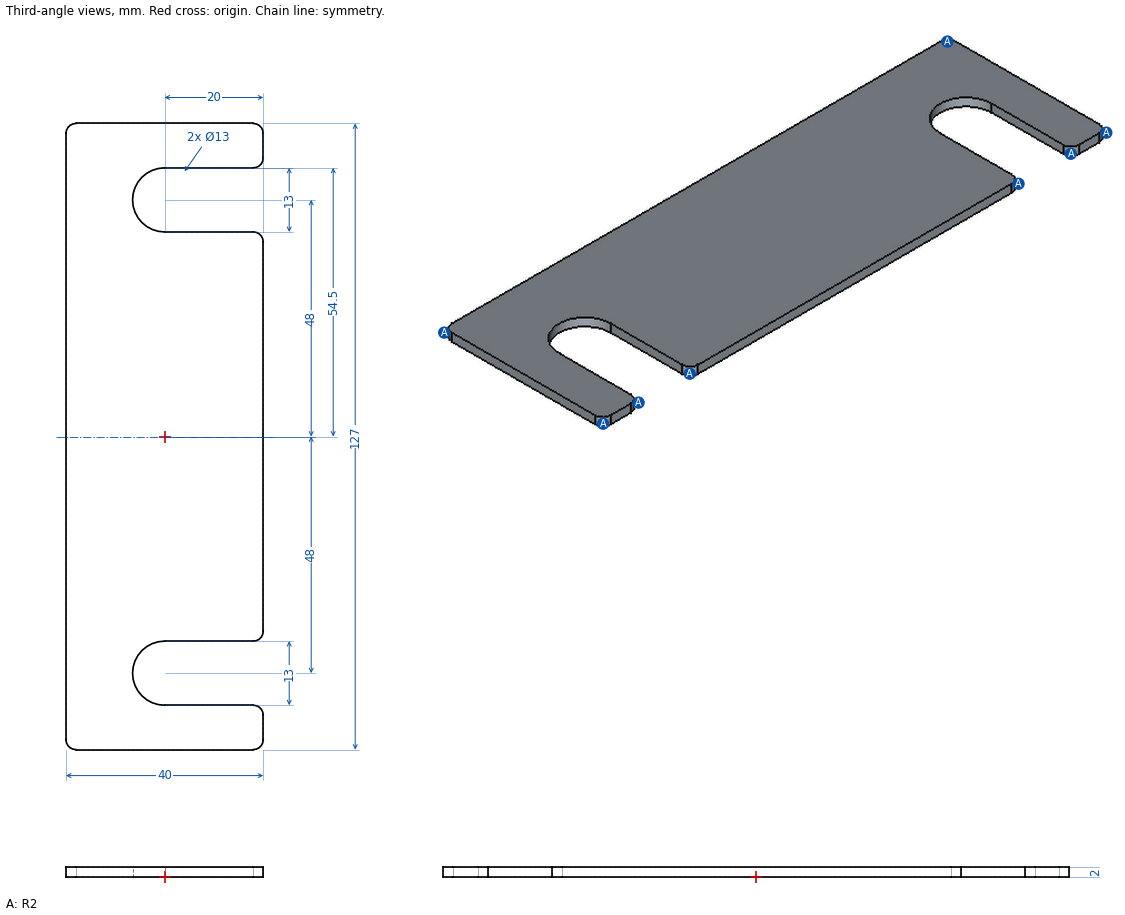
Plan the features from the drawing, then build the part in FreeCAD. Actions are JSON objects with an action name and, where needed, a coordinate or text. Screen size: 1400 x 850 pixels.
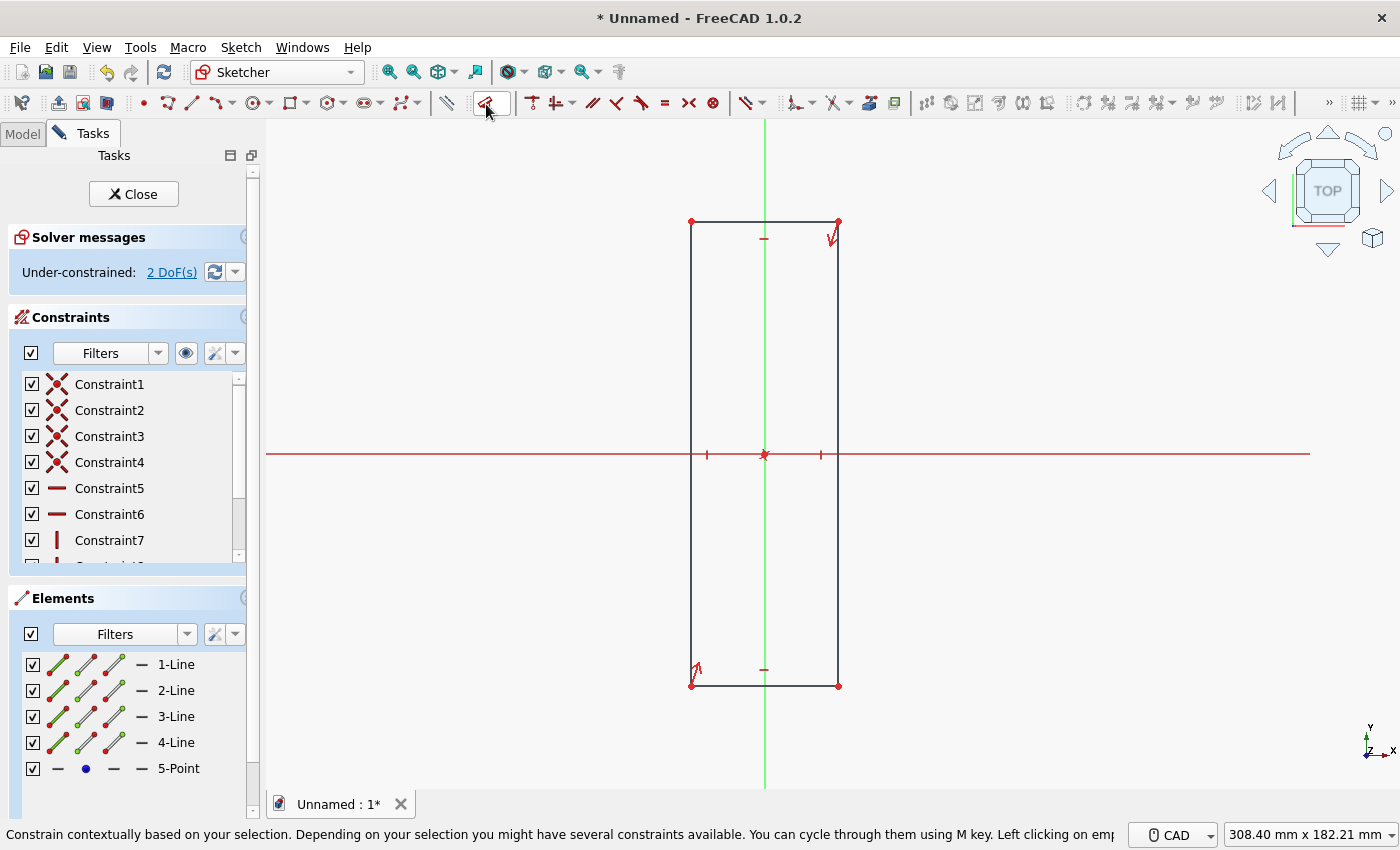
{"action": "left_click", "coordinate": [735, 686]}
{"action": "left_click", "coordinate": [731, 720]}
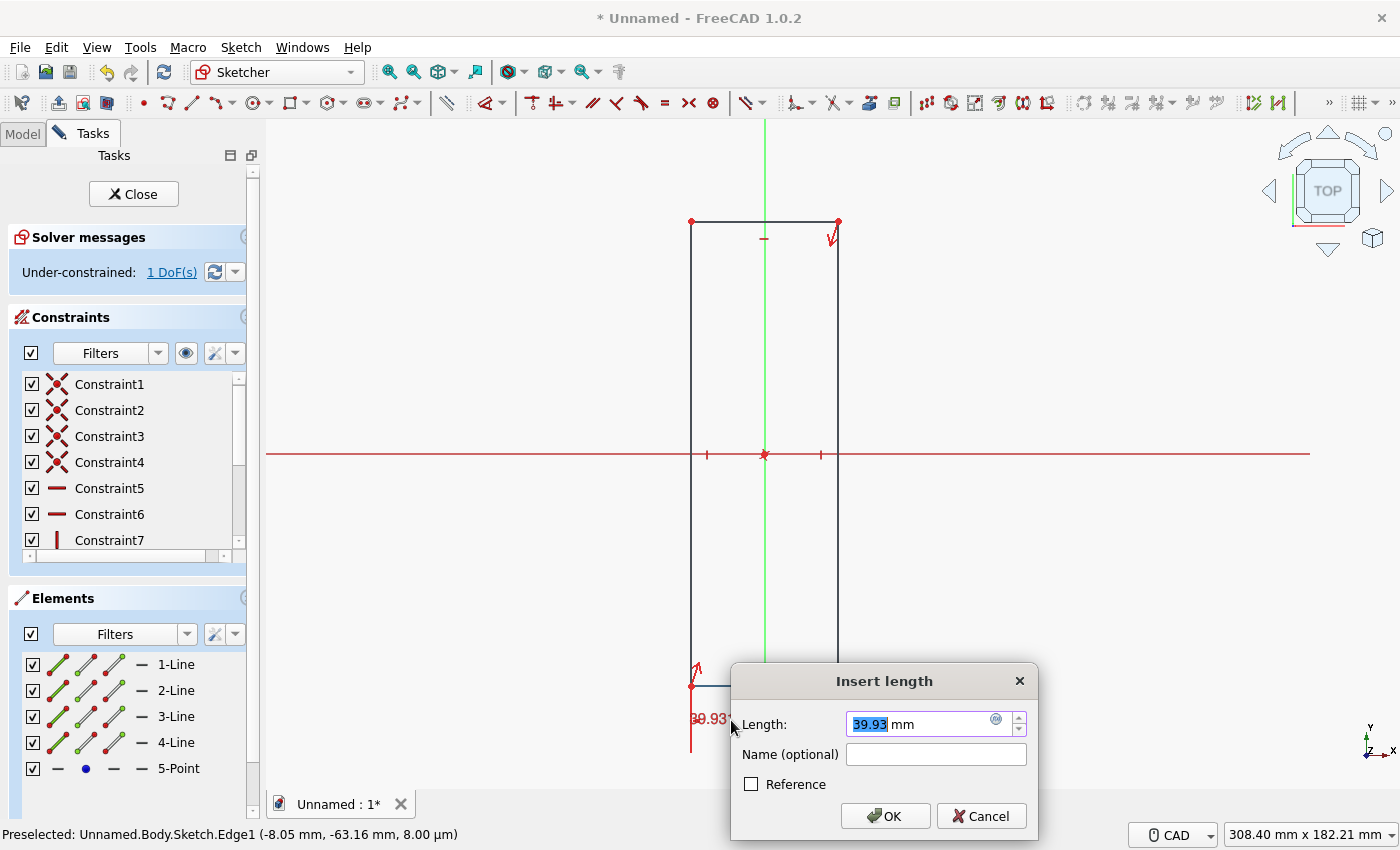
{"action": "type", "text": "40"}
{"action": "key", "text": "Return"}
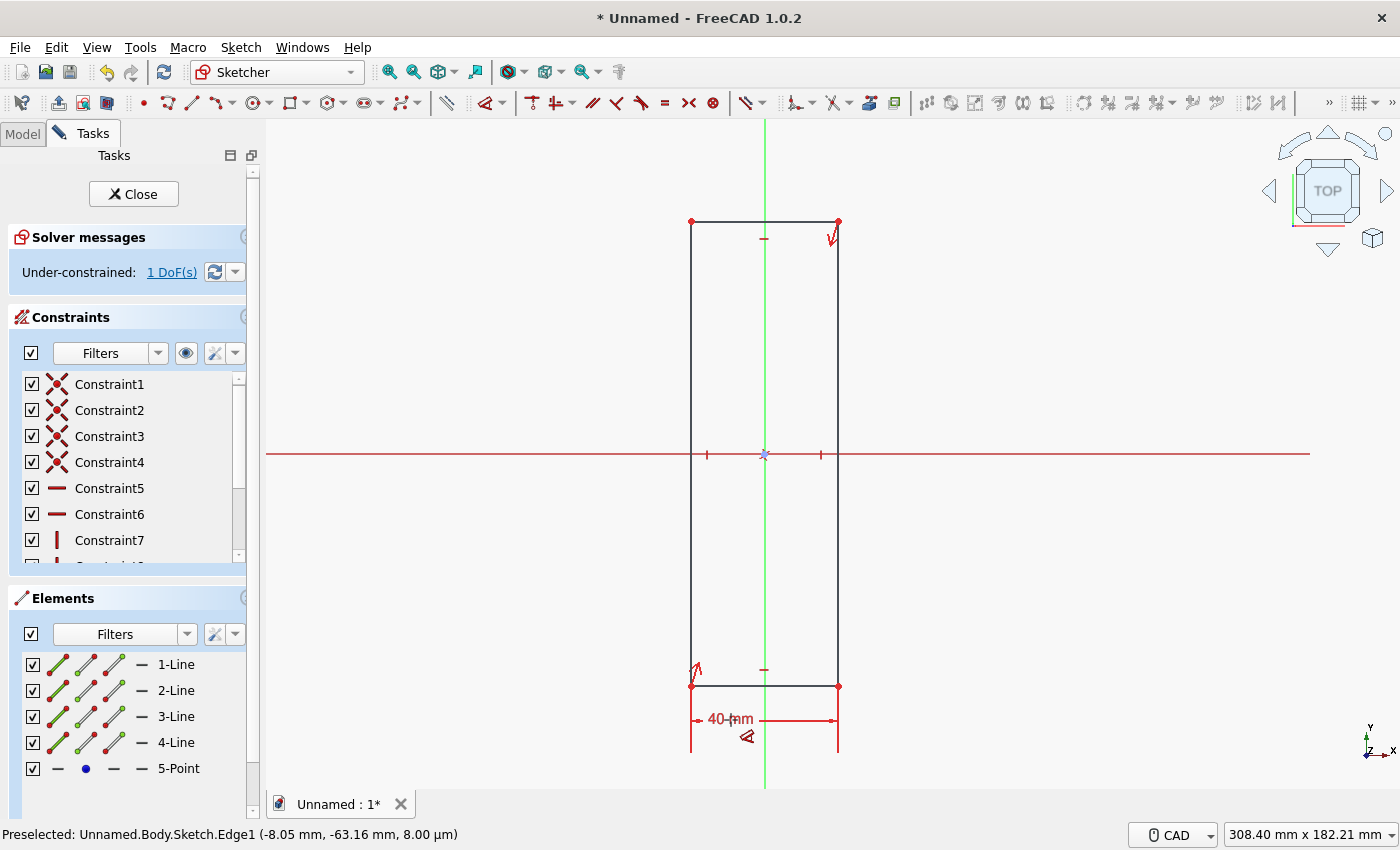
{"action": "left_click", "coordinate": [838, 547]}
{"action": "left_click", "coordinate": [872, 347]}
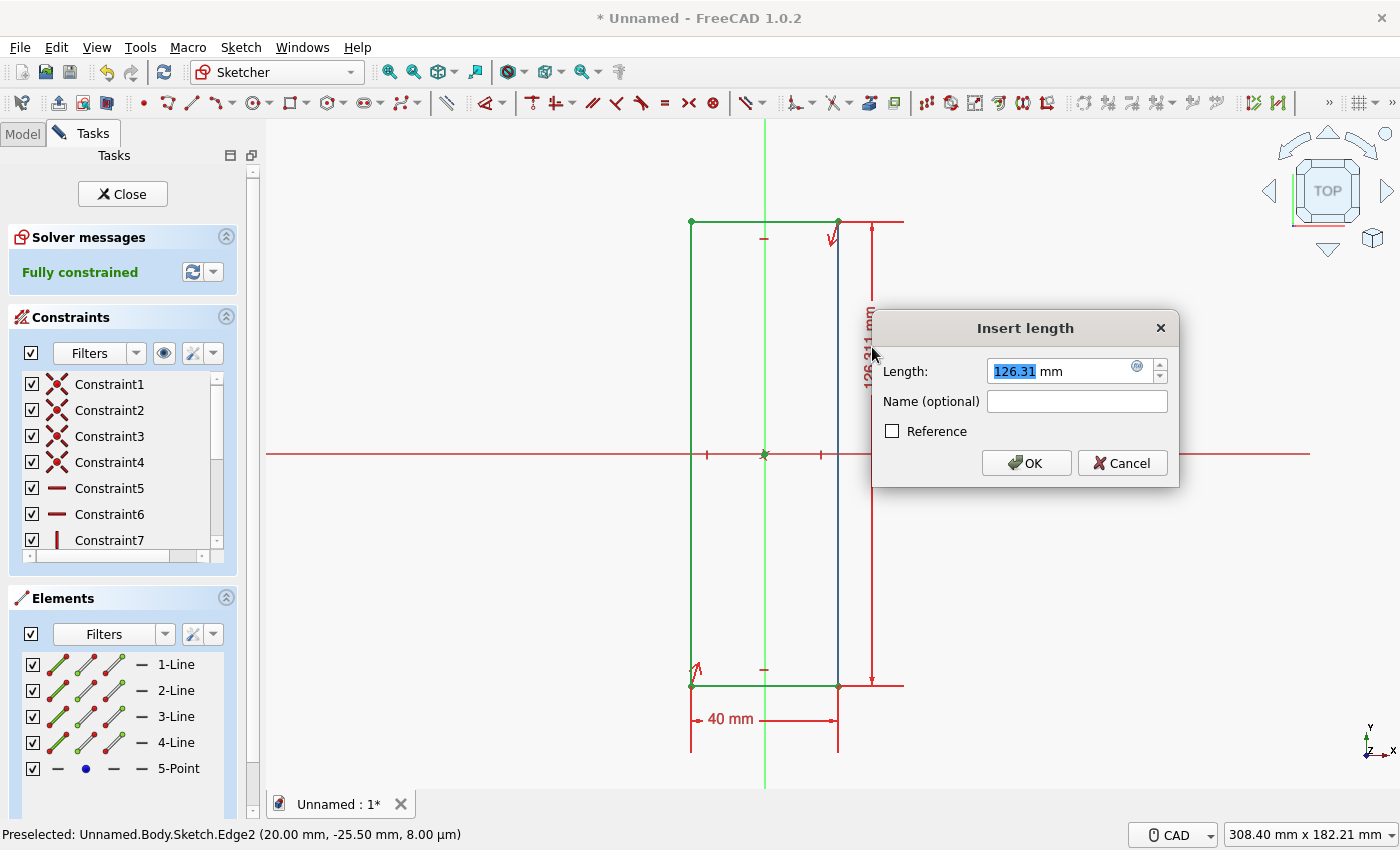
{"action": "type", "text": "127"}
{"action": "key", "text": "Return"}
{"action": "key", "text": "Escape"}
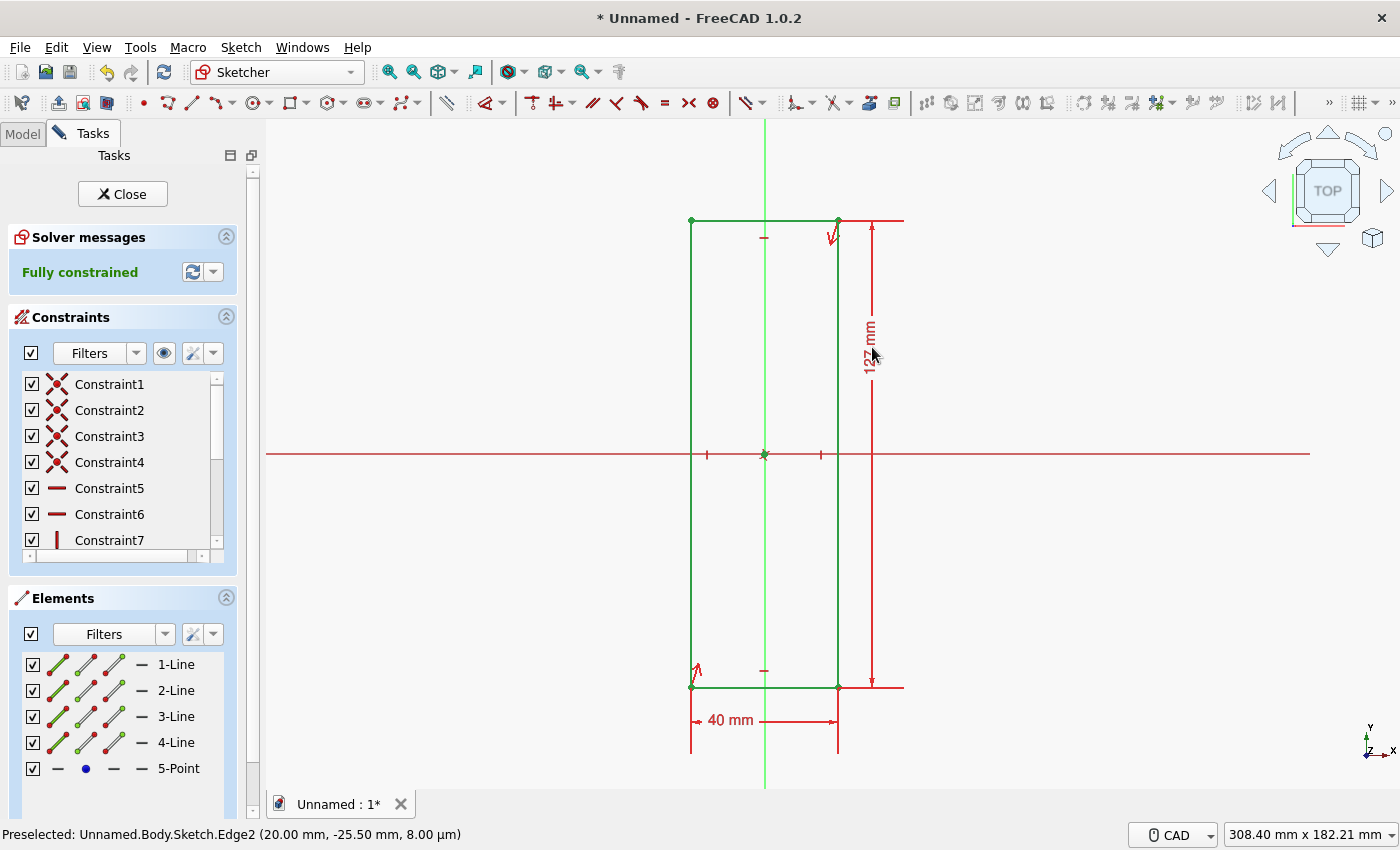
{"action": "left_click", "coordinate": [123, 194]}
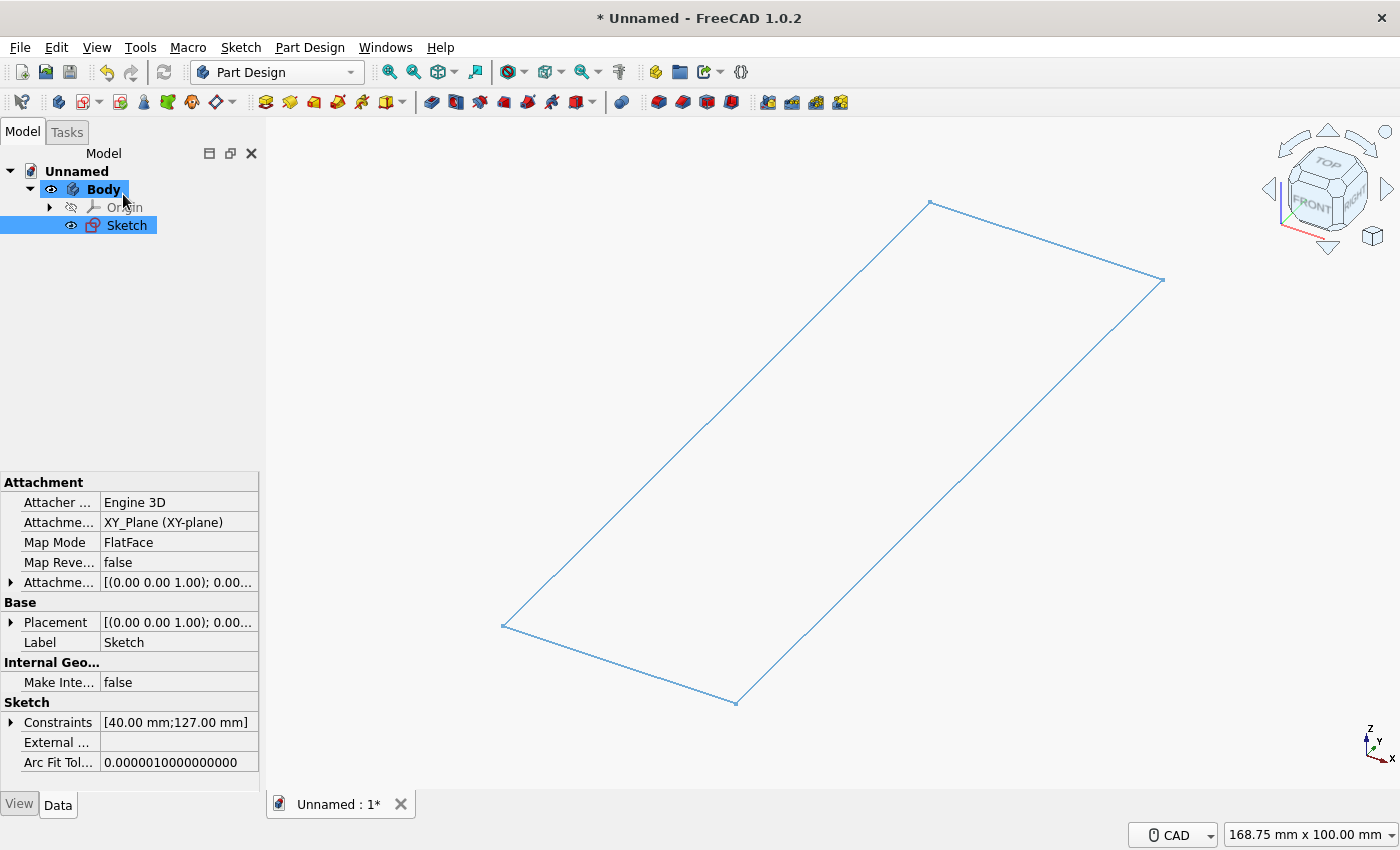
{"action": "left_click", "coordinate": [266, 102]}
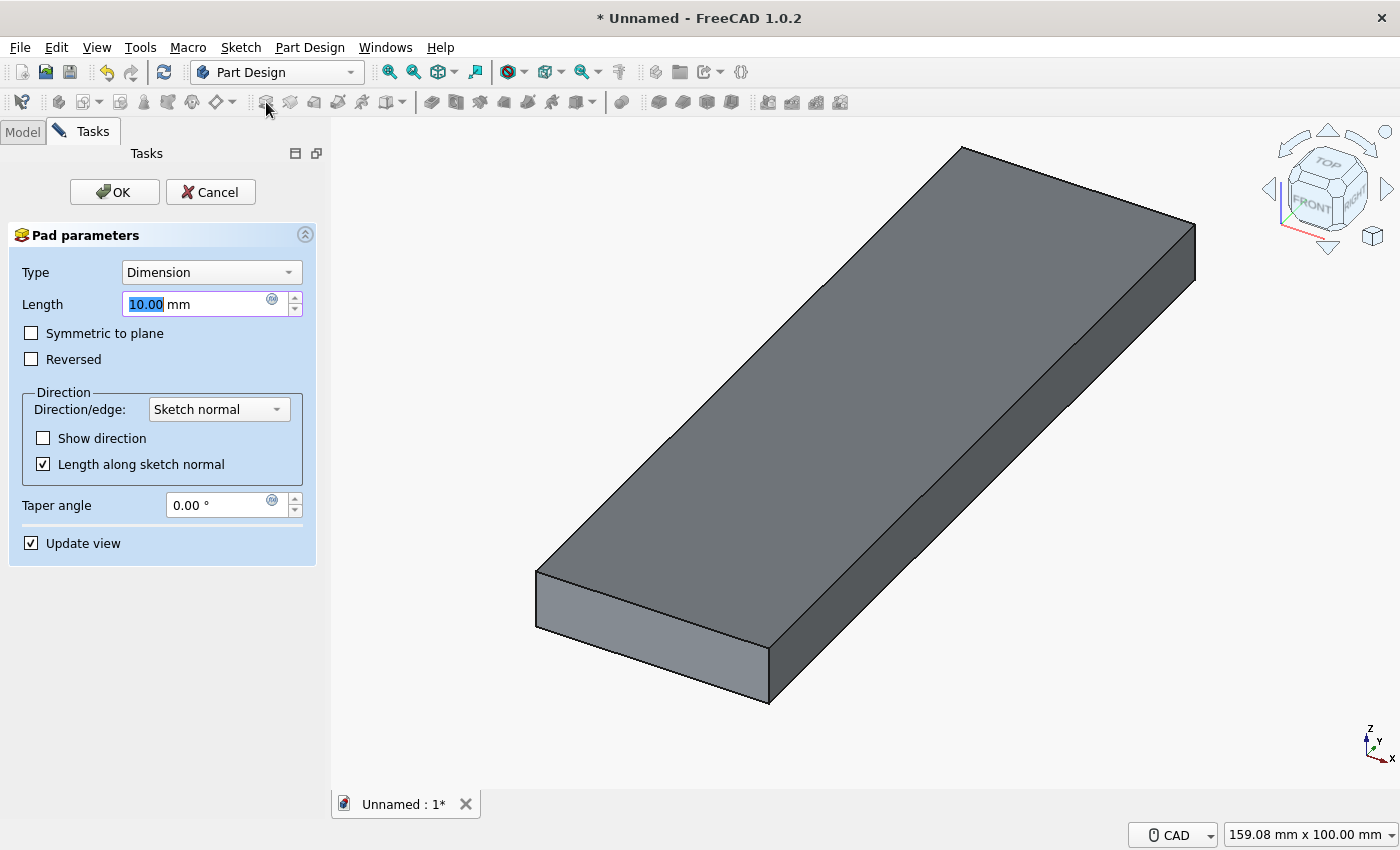
{"action": "type", "text": "2"}
{"action": "key", "text": "Tab"}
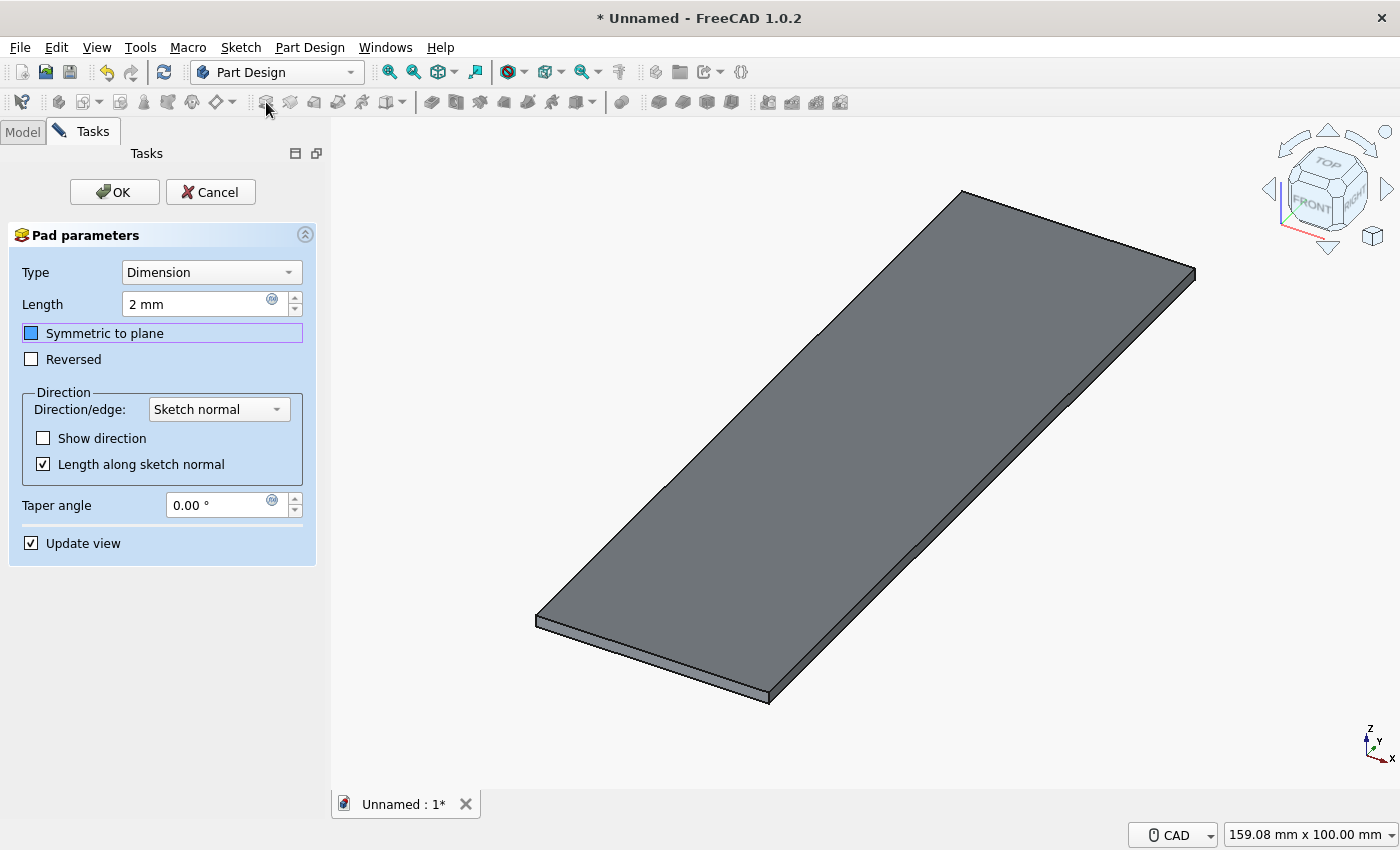
{"action": "left_click", "coordinate": [115, 192]}